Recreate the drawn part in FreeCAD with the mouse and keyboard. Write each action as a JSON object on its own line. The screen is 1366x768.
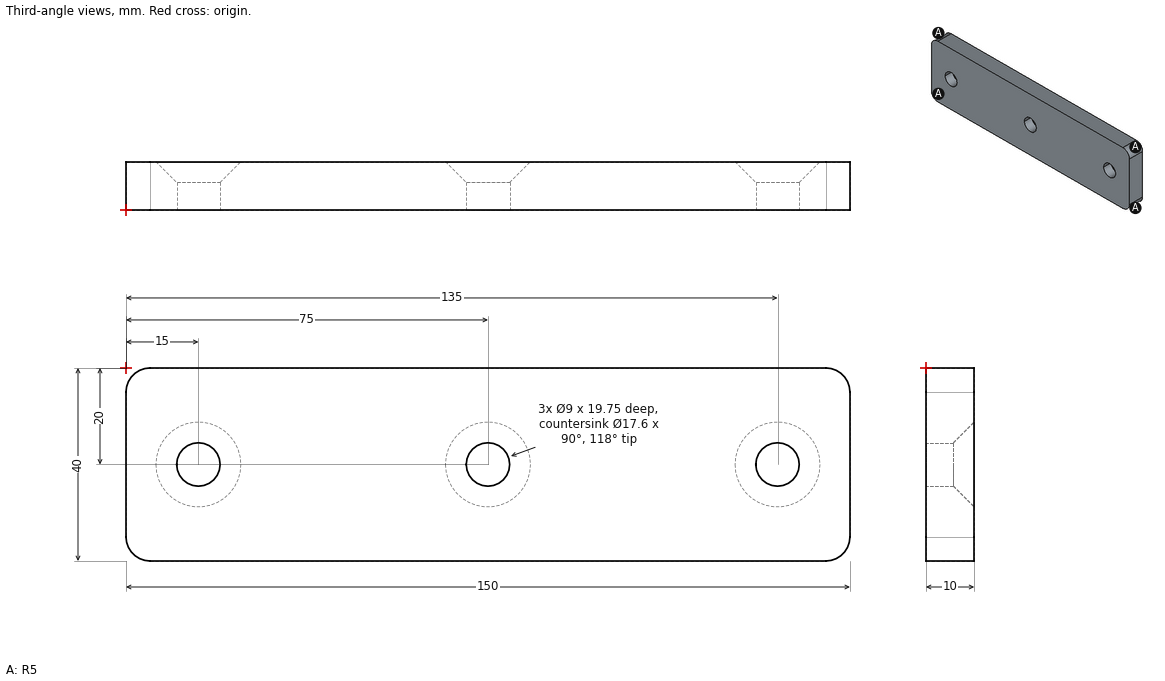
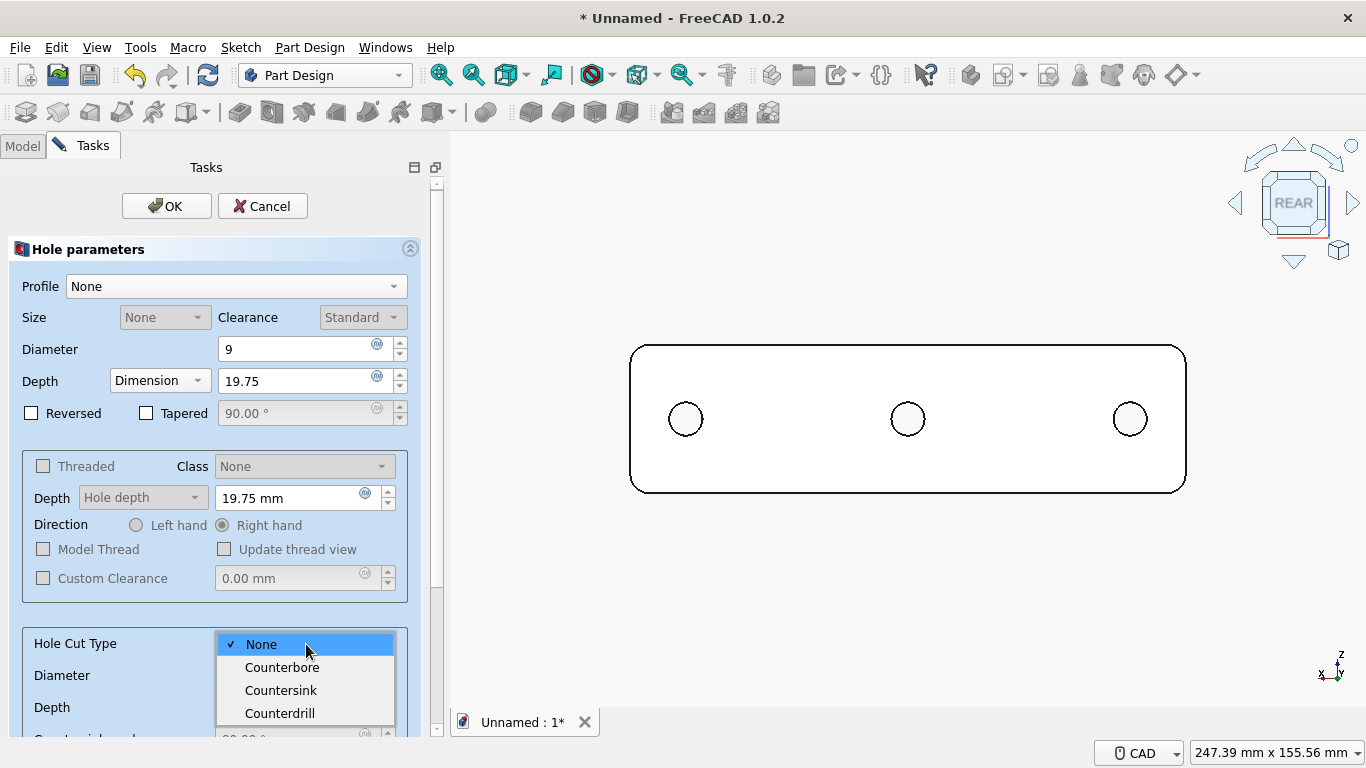
{"action": "left_click", "coordinate": [304, 690]}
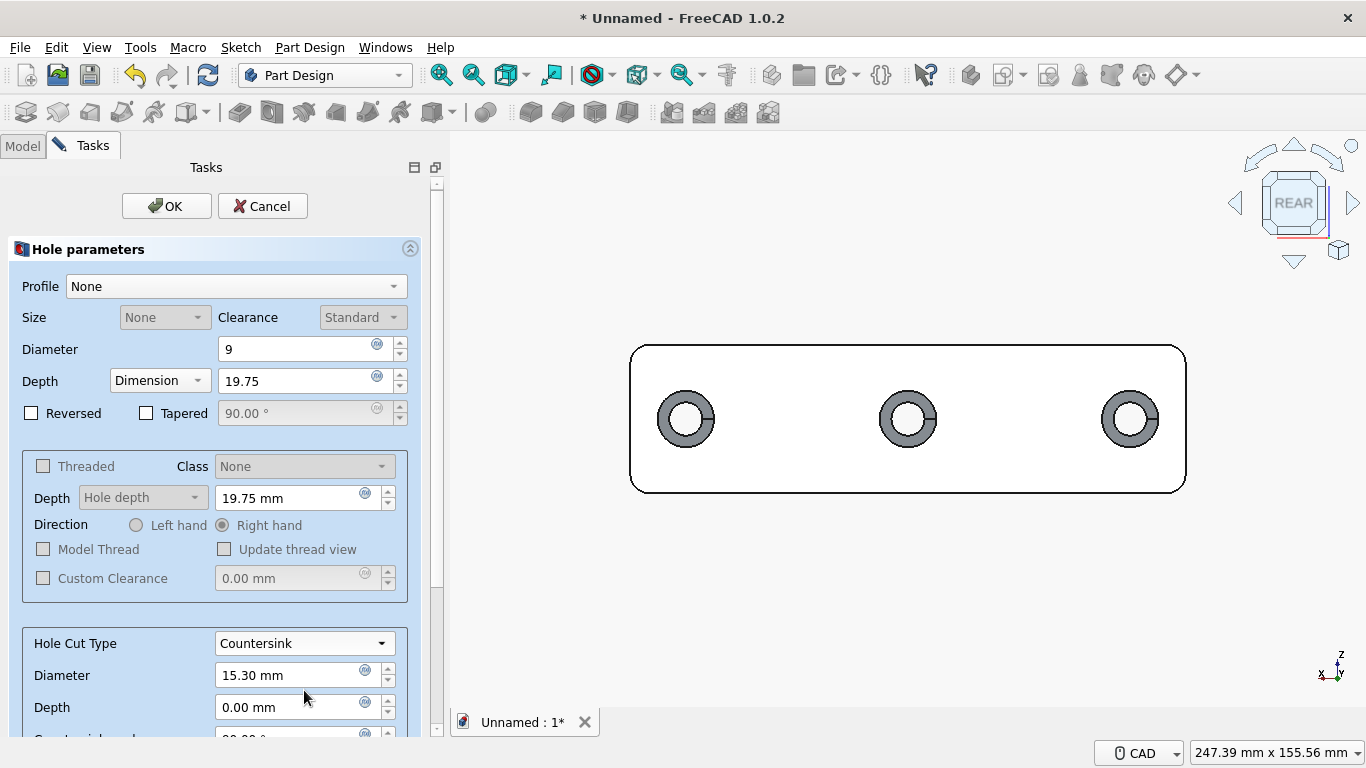
{"action": "triple_click", "coordinate": [298, 675]}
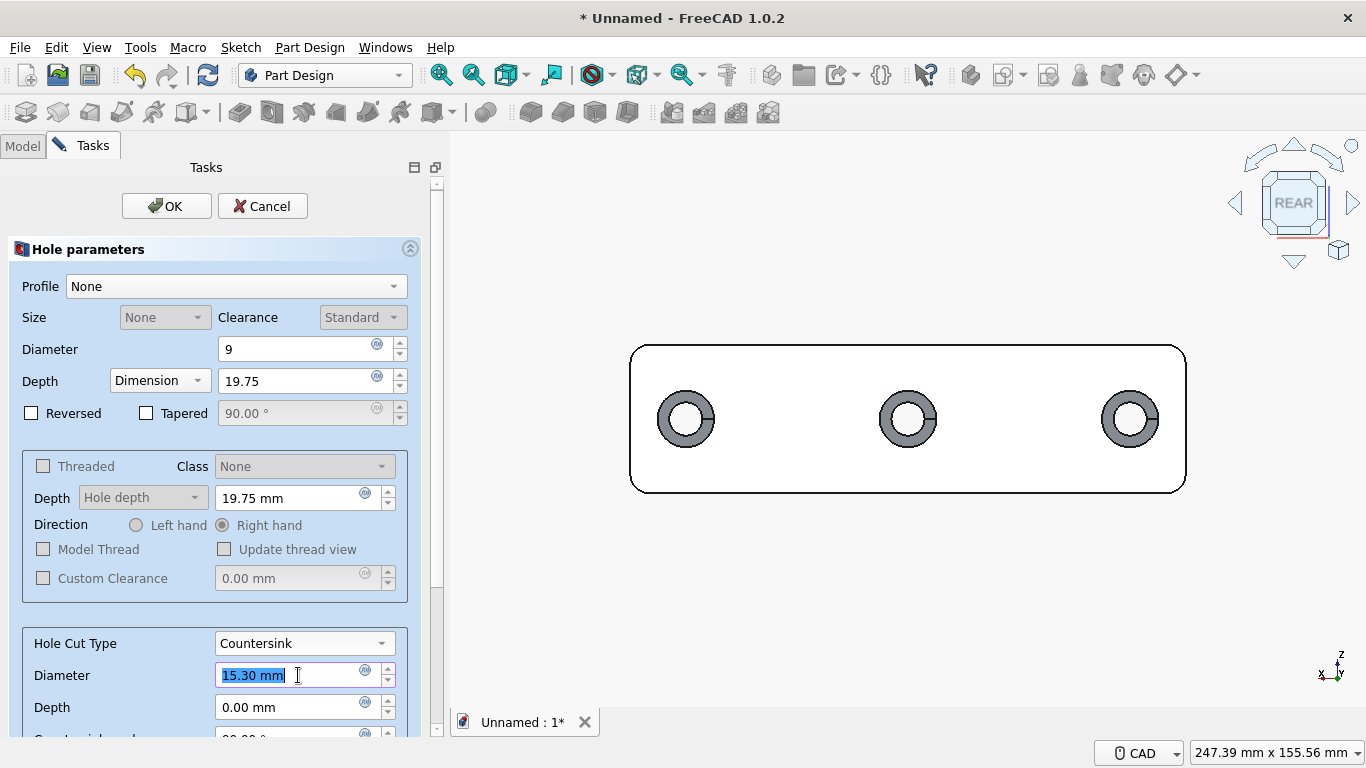
{"action": "type", "text": "17.6"}
{"action": "key", "text": "Tab"}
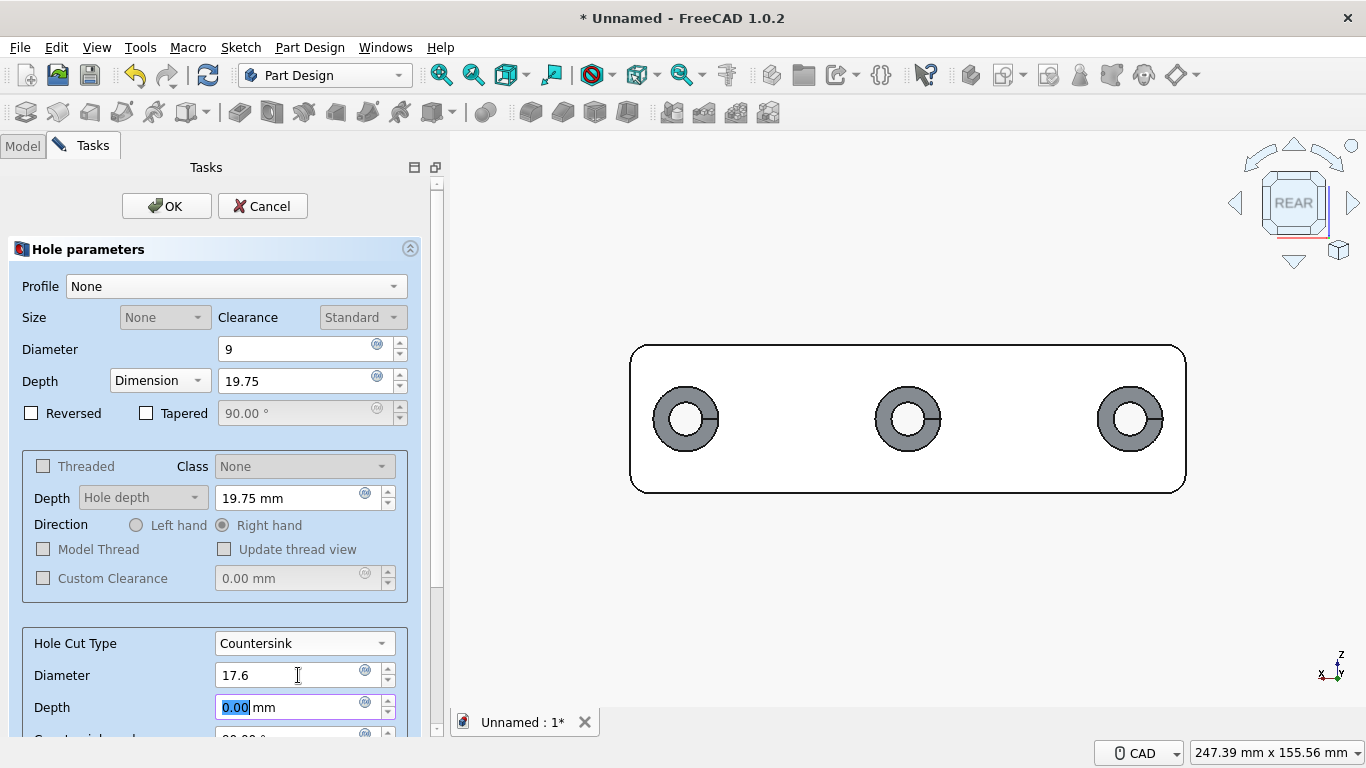
{"action": "left_click", "coordinate": [167, 206]}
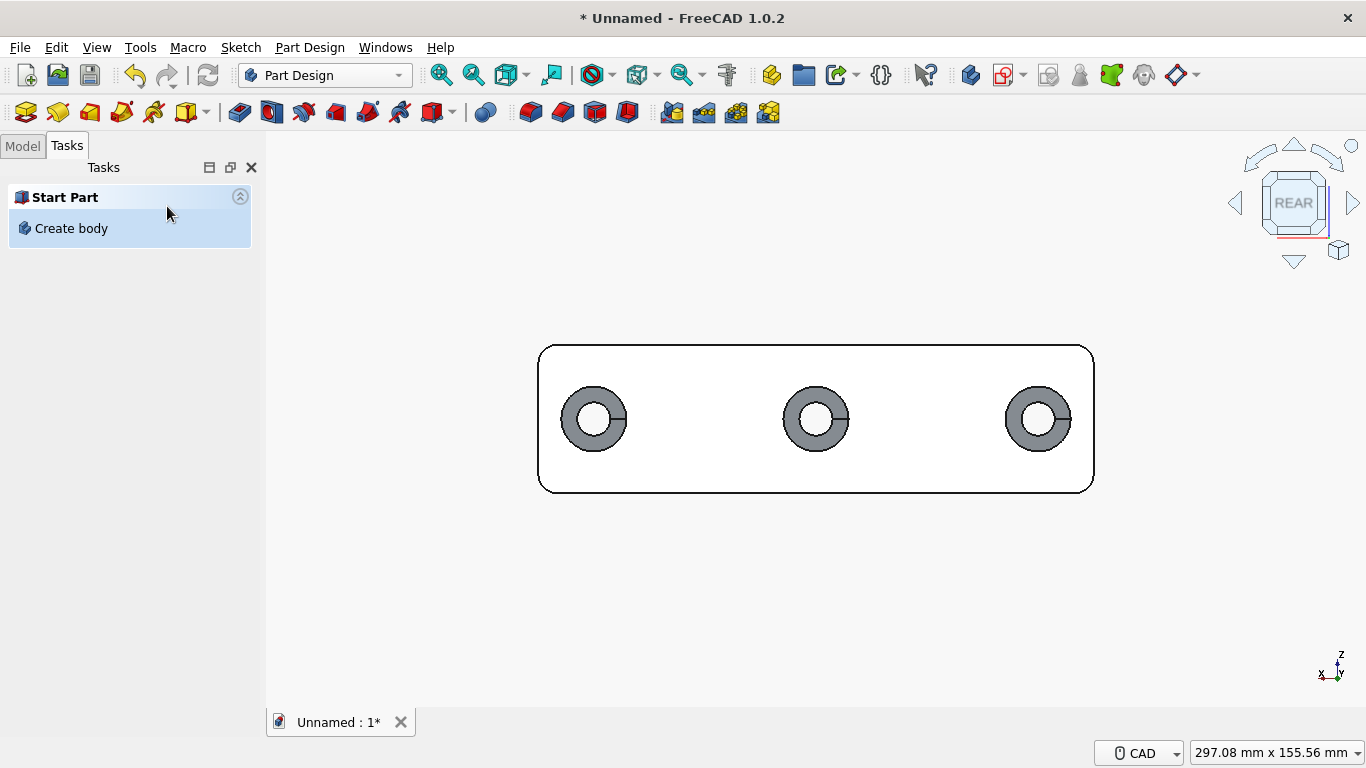
{"action": "key", "text": "0"}